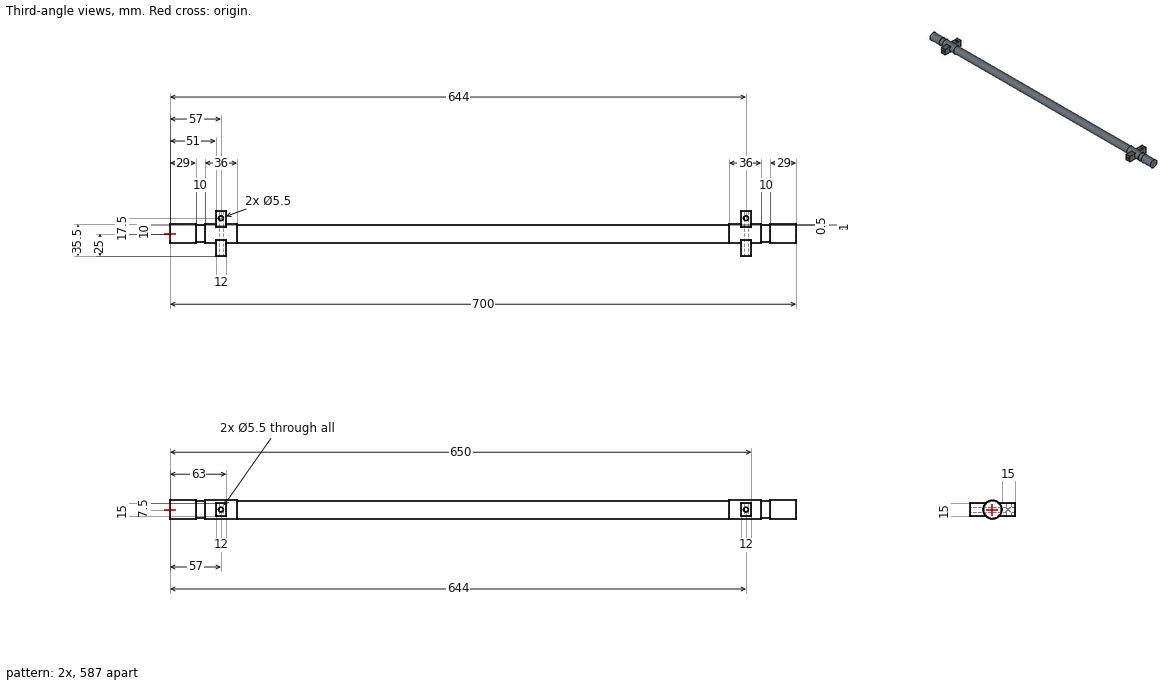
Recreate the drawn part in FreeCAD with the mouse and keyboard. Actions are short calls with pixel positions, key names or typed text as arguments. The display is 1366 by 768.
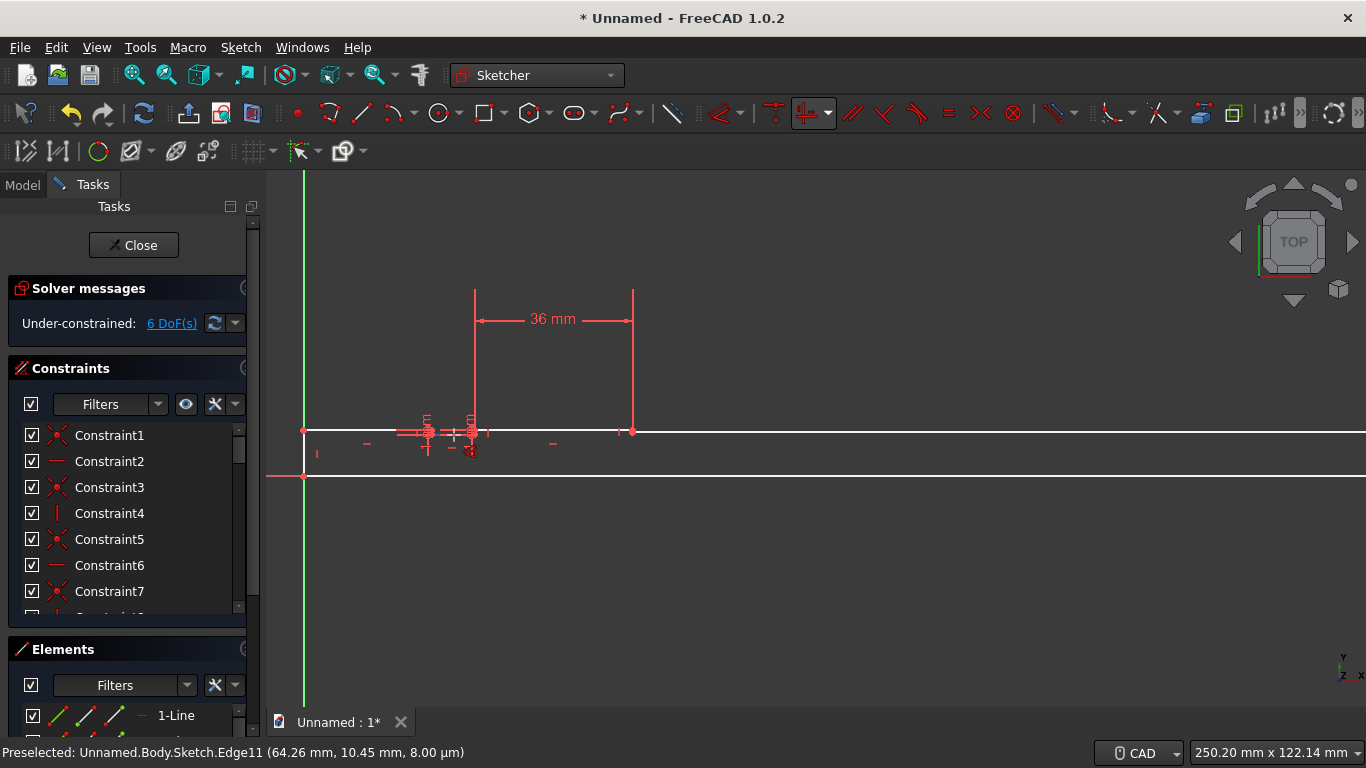
click(453, 435)
click(453, 401)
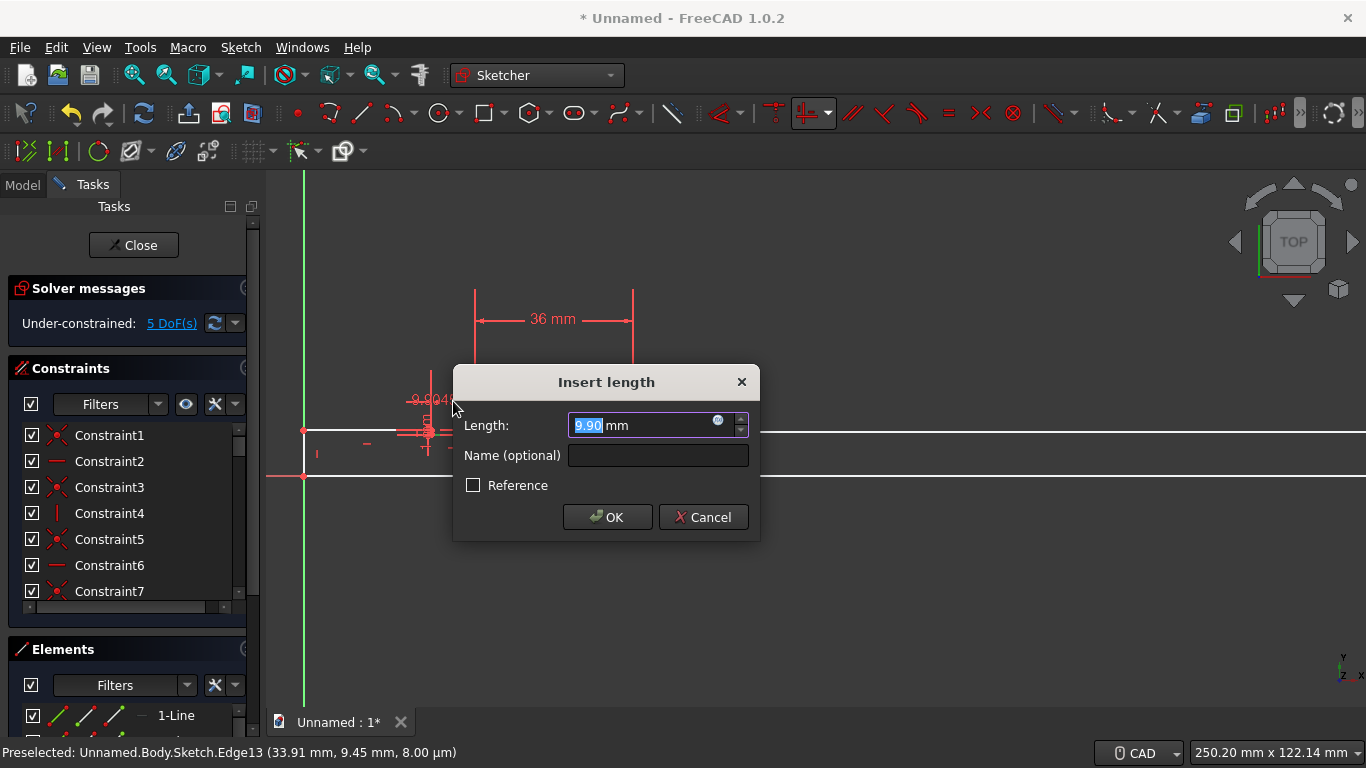
text(10)
key(Return)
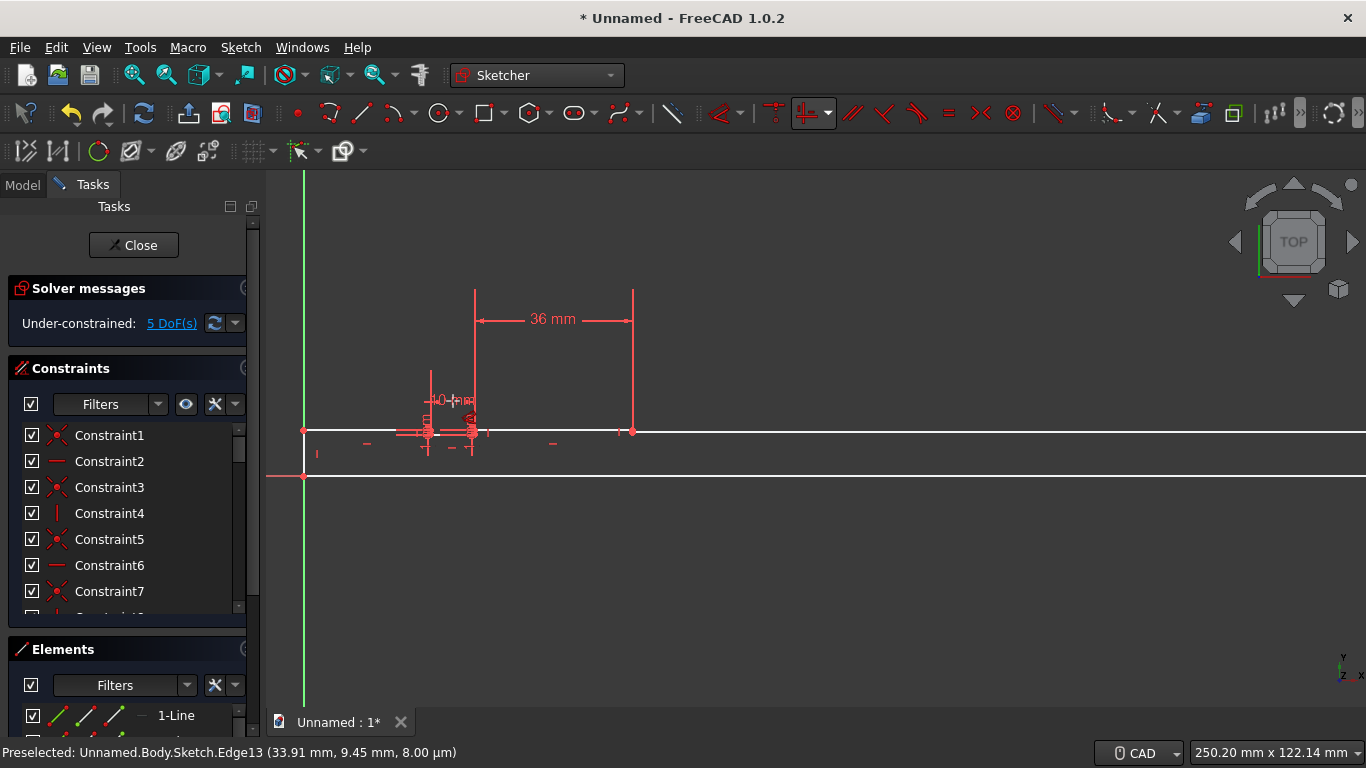
click(393, 430)
click(367, 396)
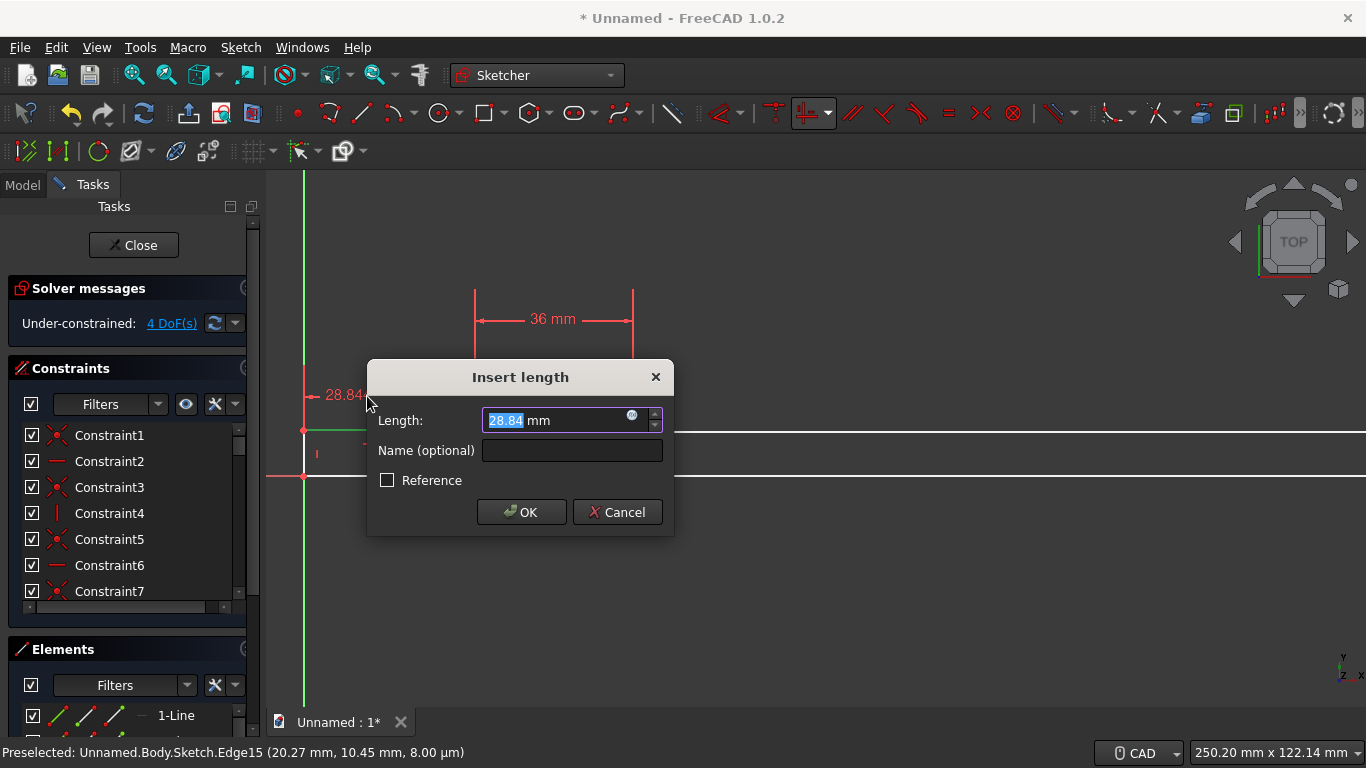
text(29)
key(Return)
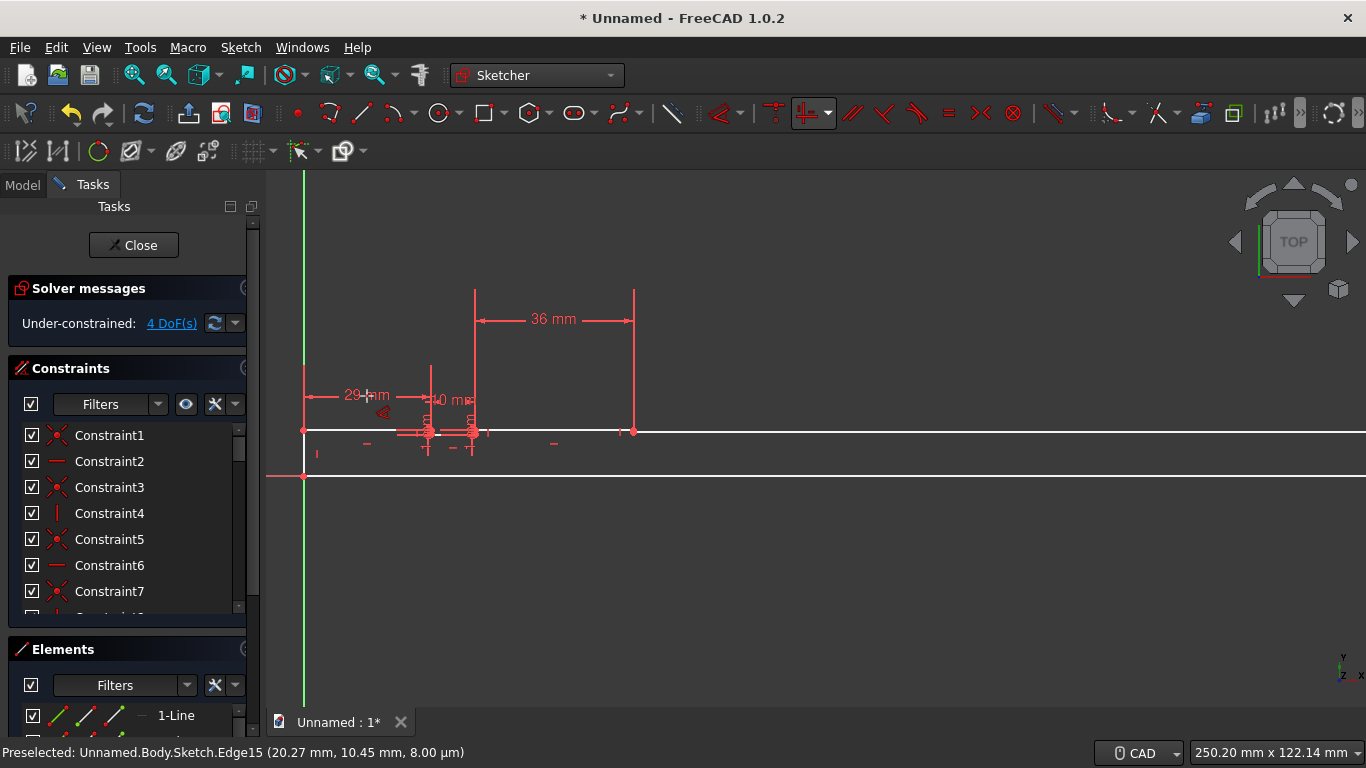
scroll(470, 435, down, 8)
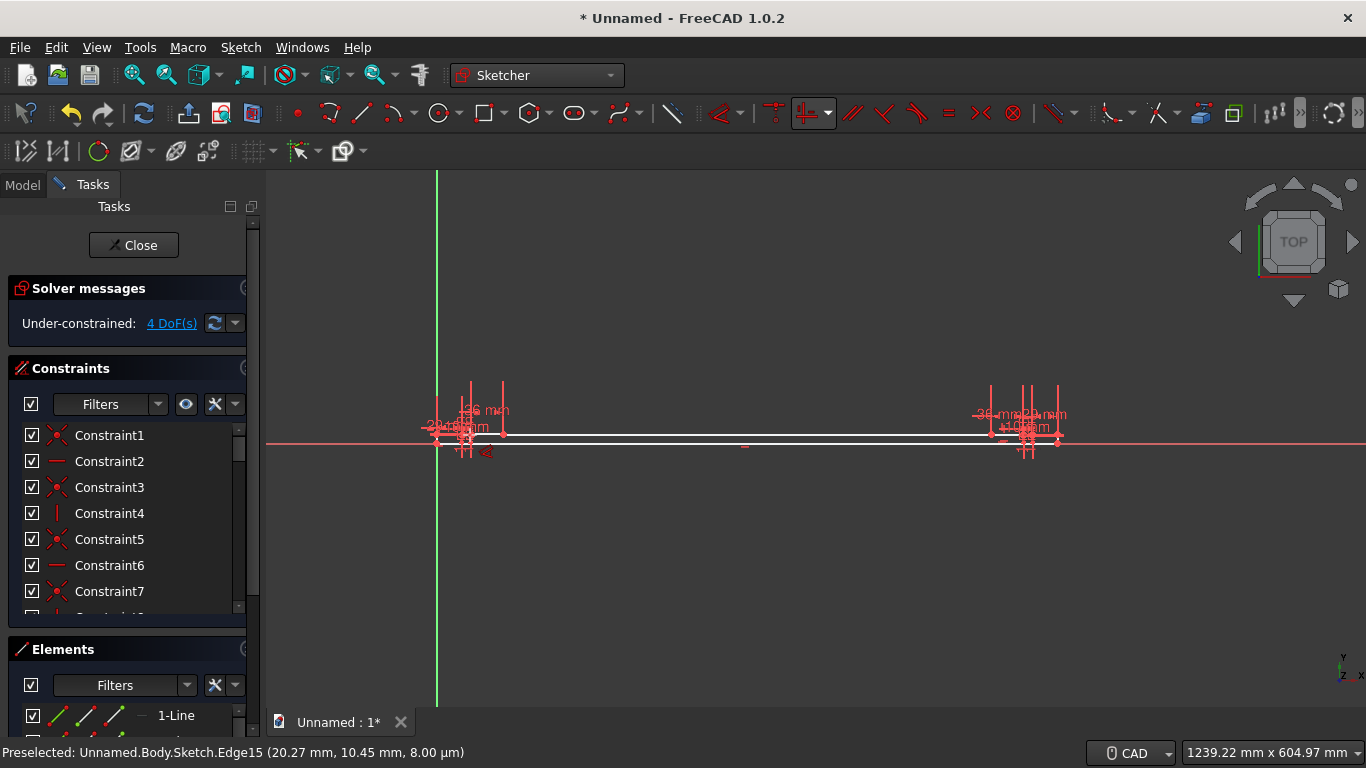
scroll(561, 444, up, 3)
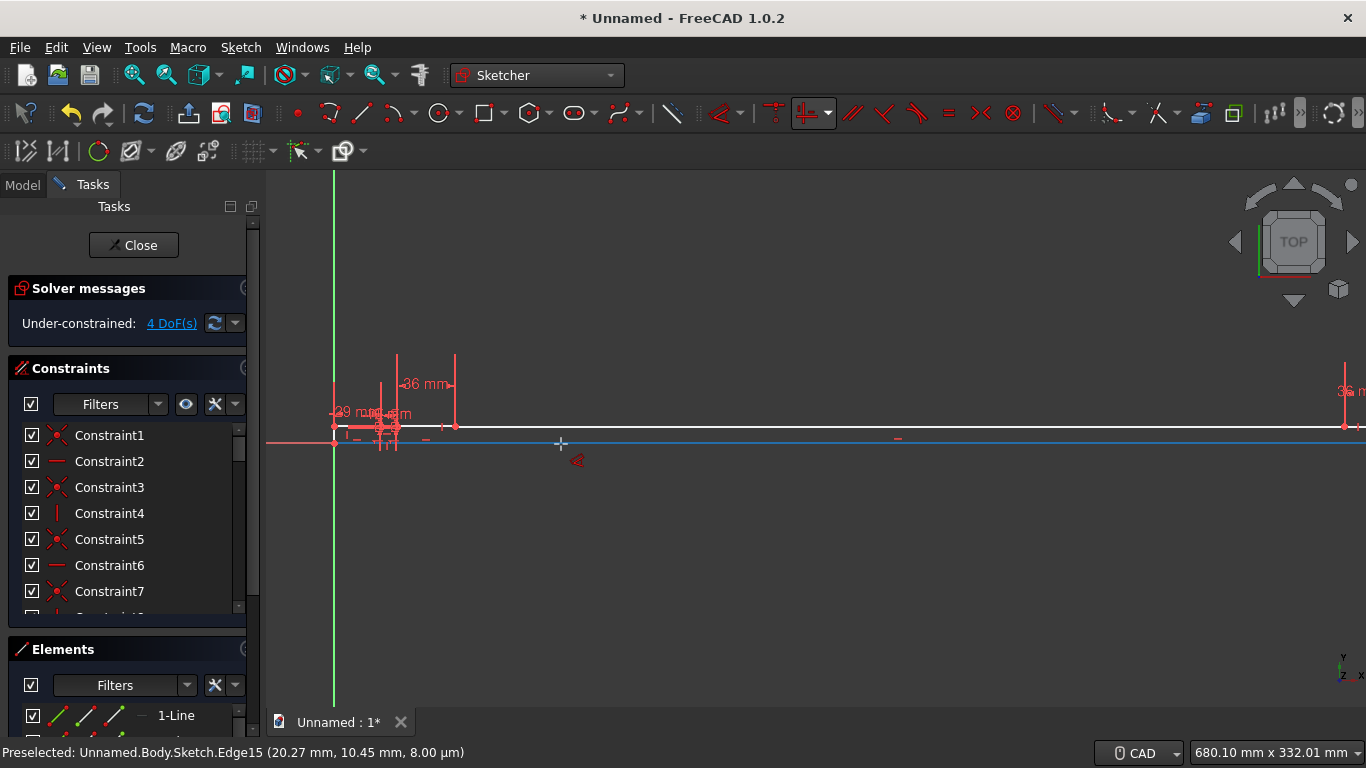
click(560, 443)
click(768, 477)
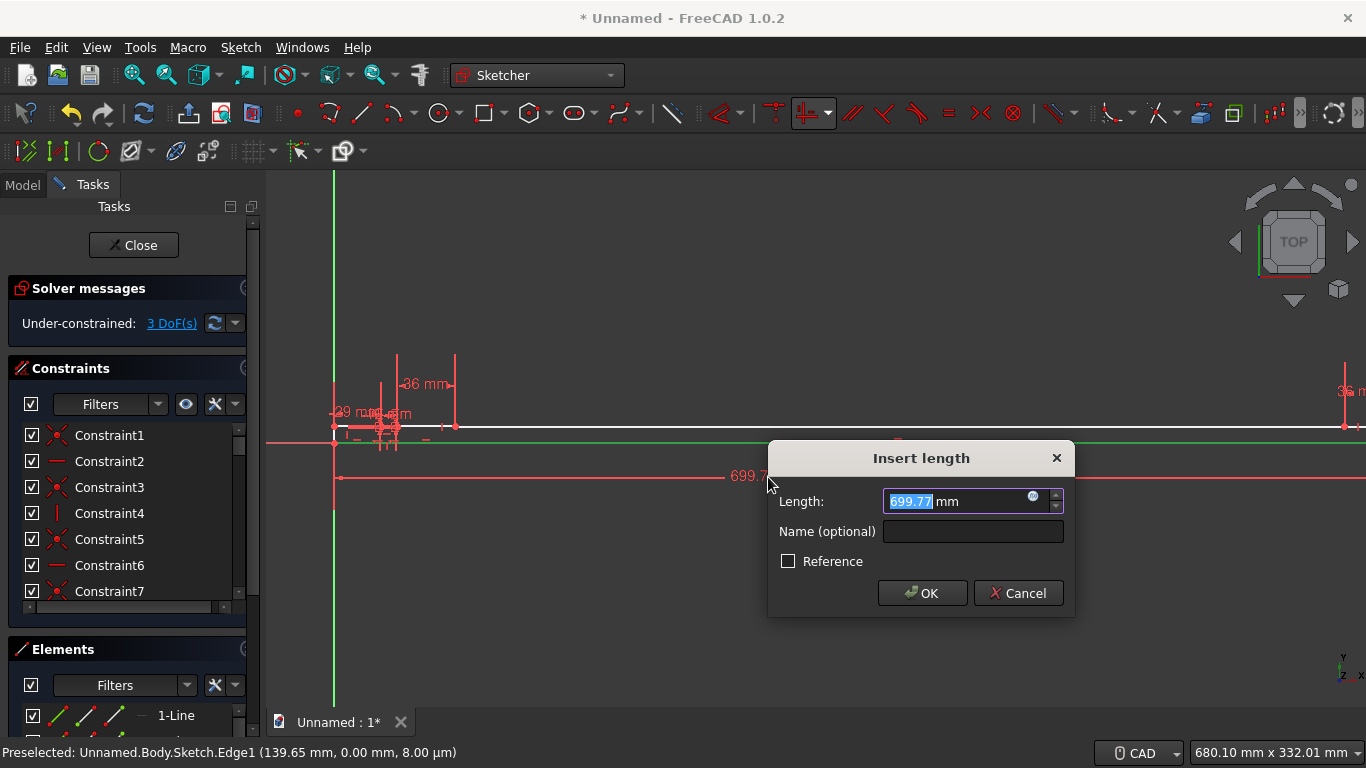
text(700)
key(Return)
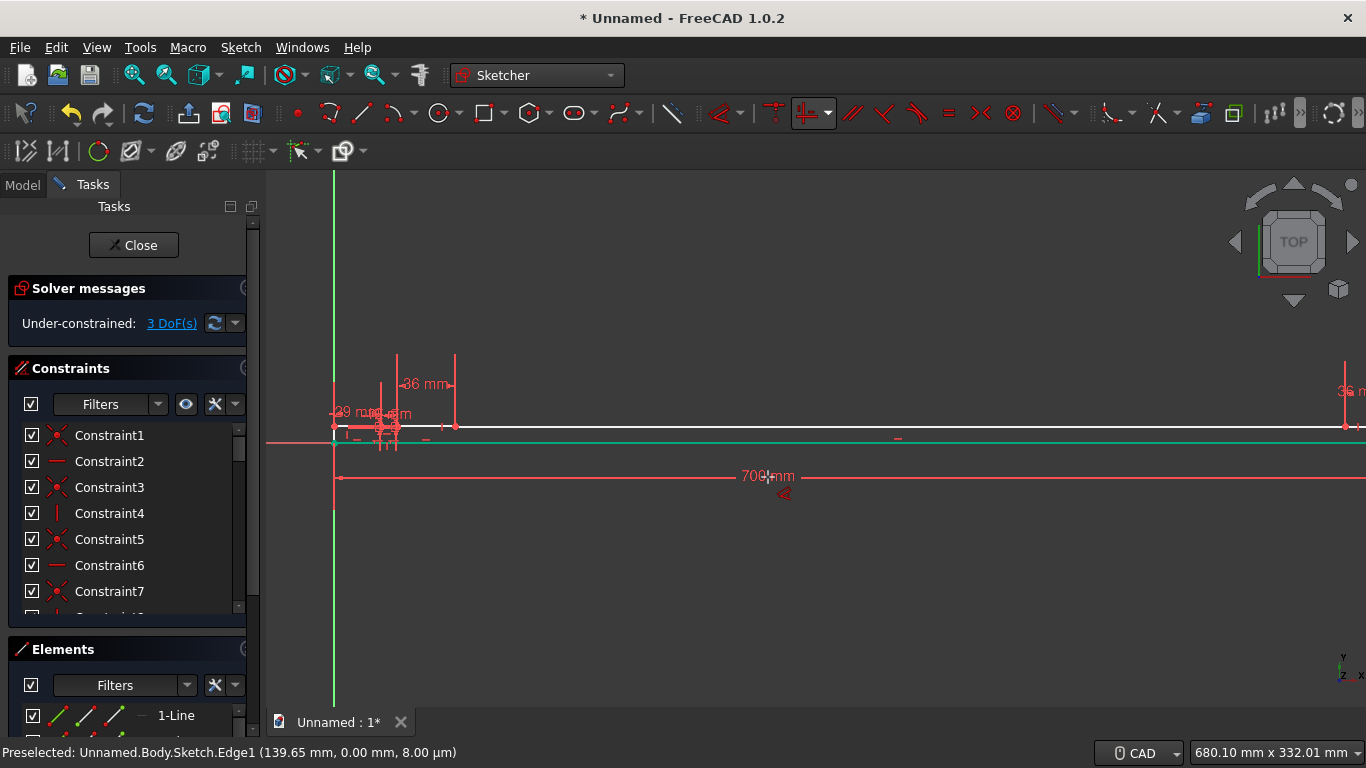
scroll(562, 443, down, 3)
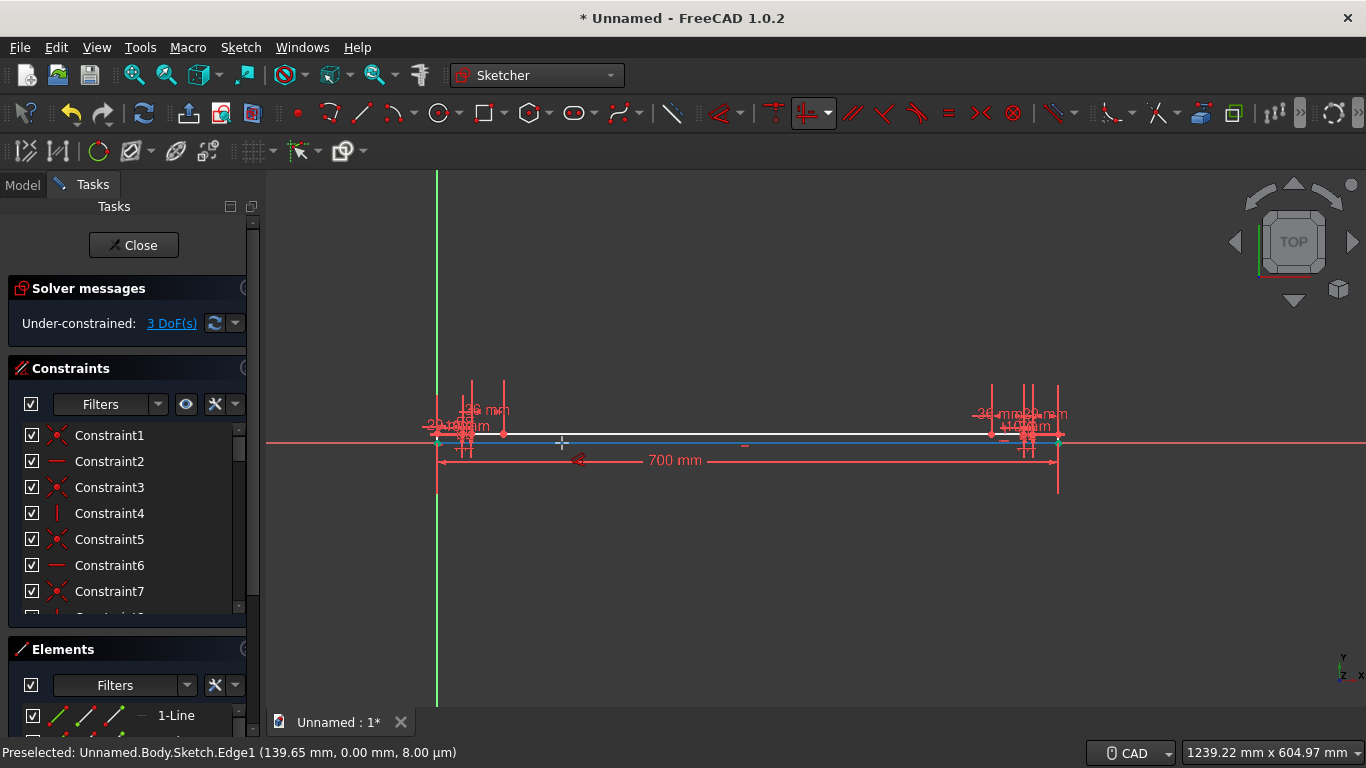
scroll(992, 434, up, 23)